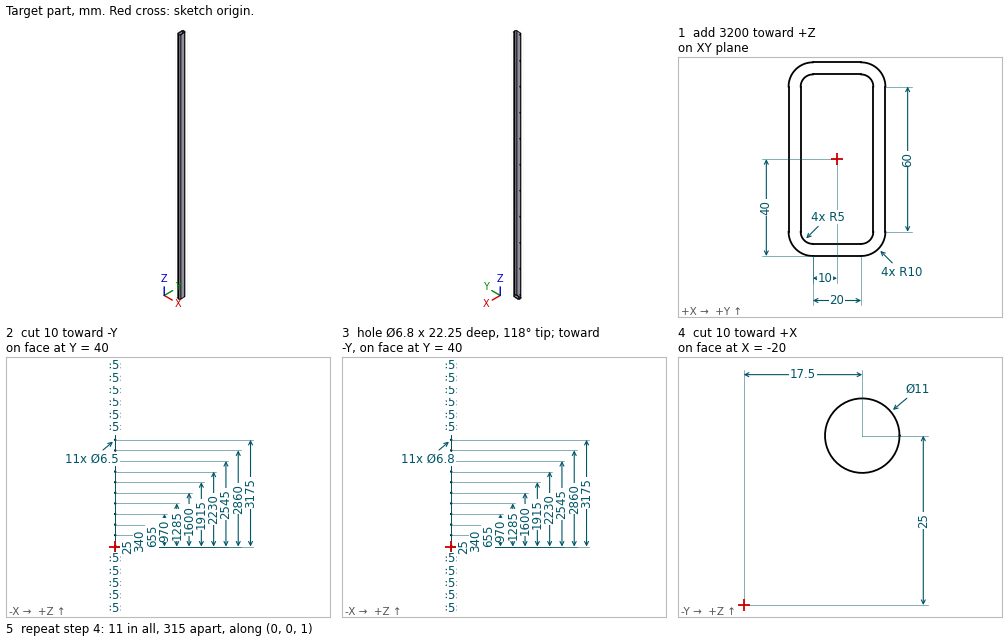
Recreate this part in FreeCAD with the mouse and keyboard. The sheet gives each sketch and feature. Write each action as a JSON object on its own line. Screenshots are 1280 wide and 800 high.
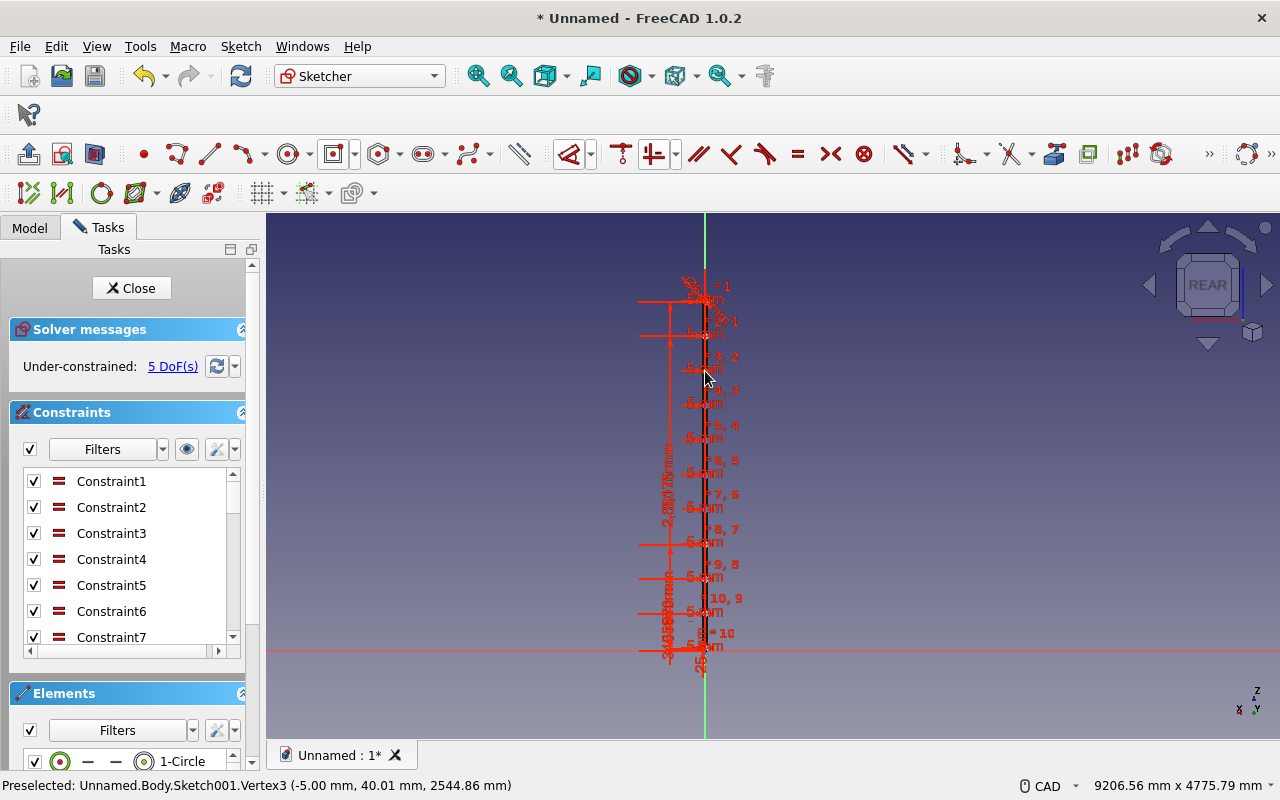
{"action": "key", "text": "i"}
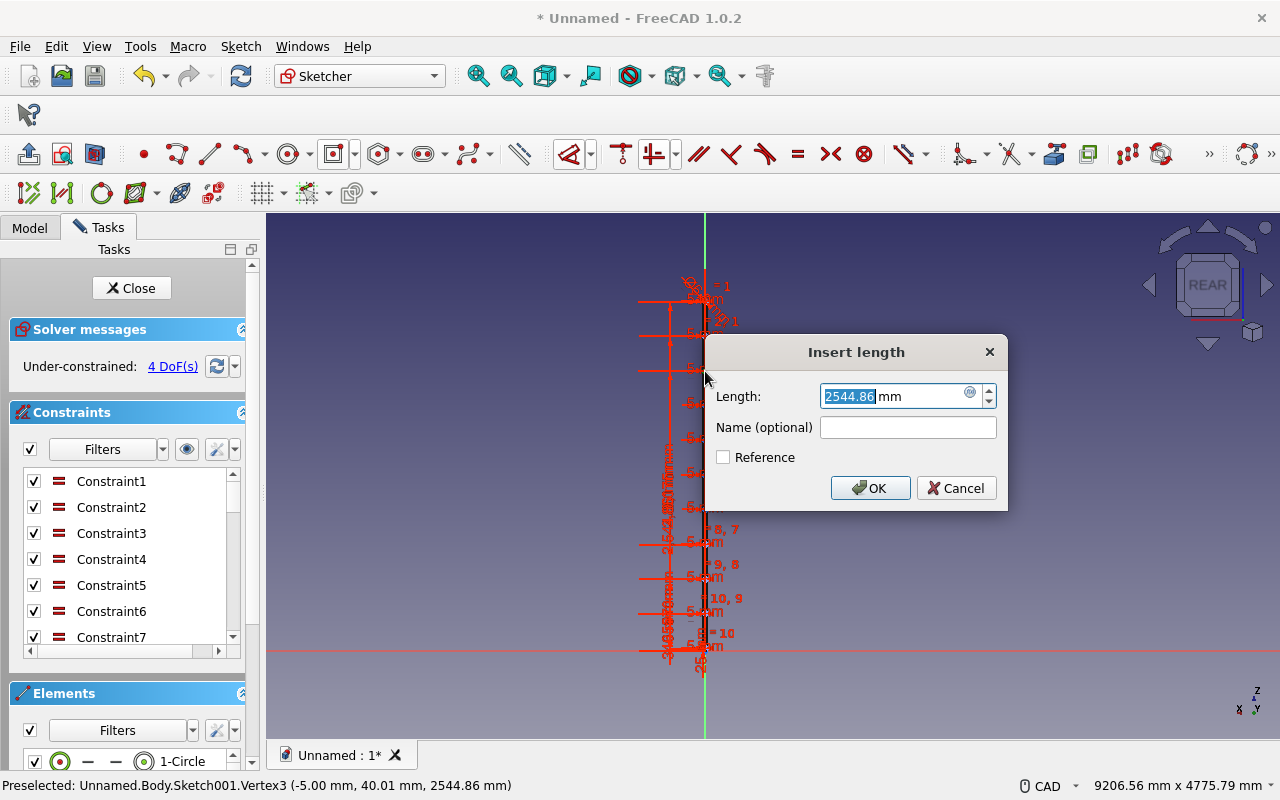
{"action": "type", "text": "2545"}
{"action": "key", "text": "Return"}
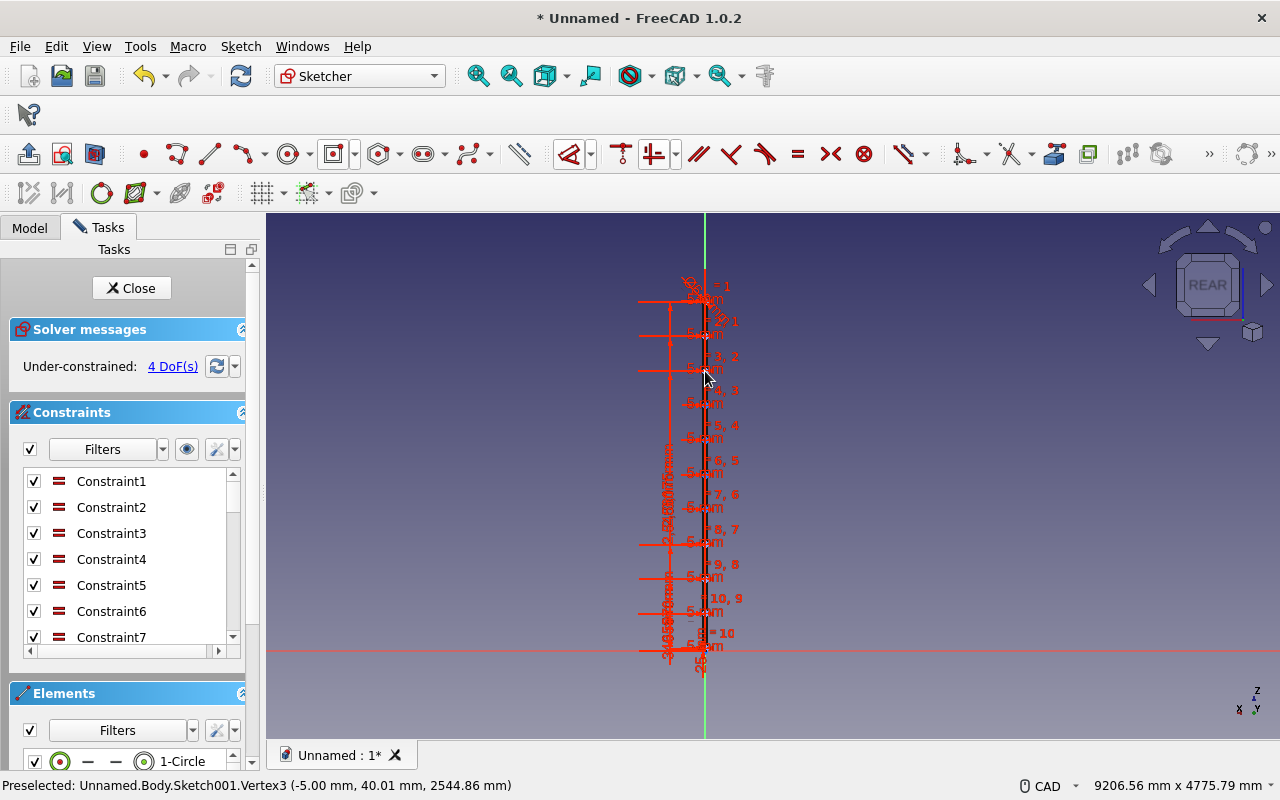
{"action": "left_click", "coordinate": [705, 406]}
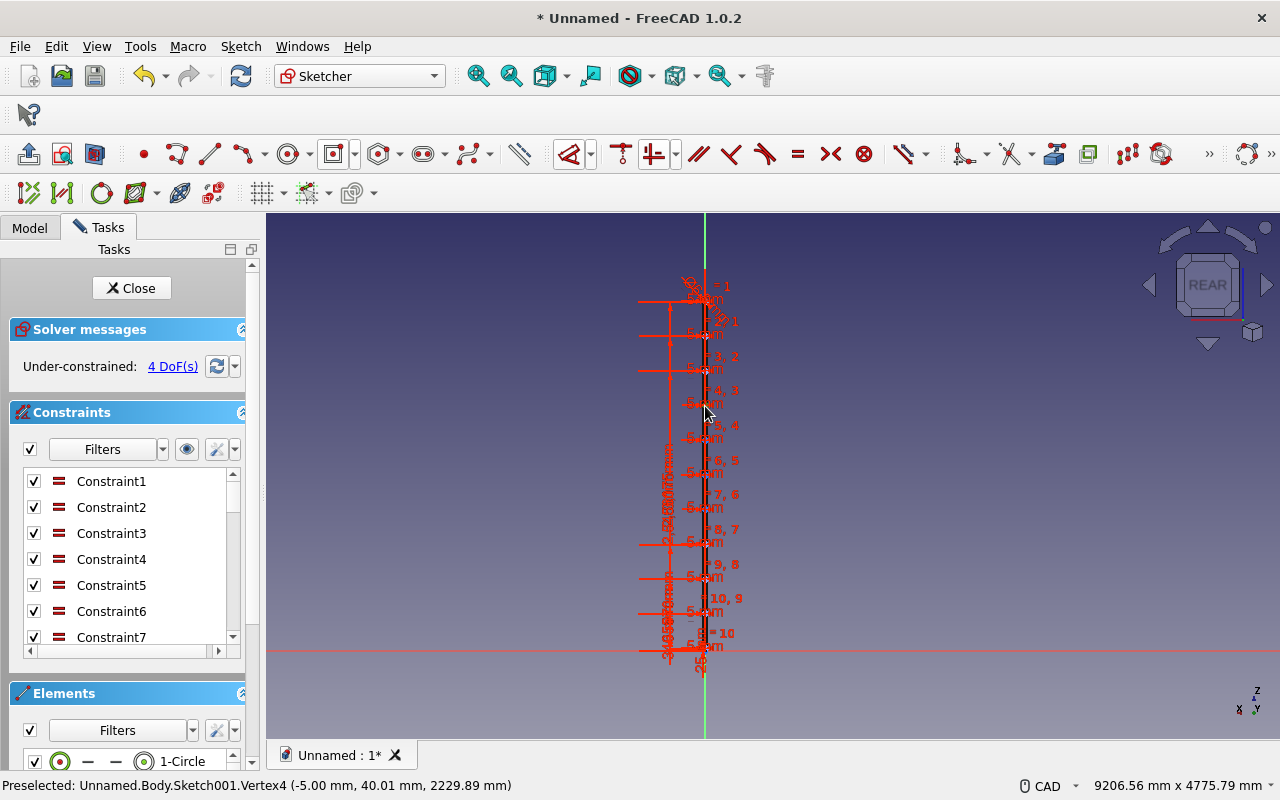
{"action": "left_click", "coordinate": [590, 154]}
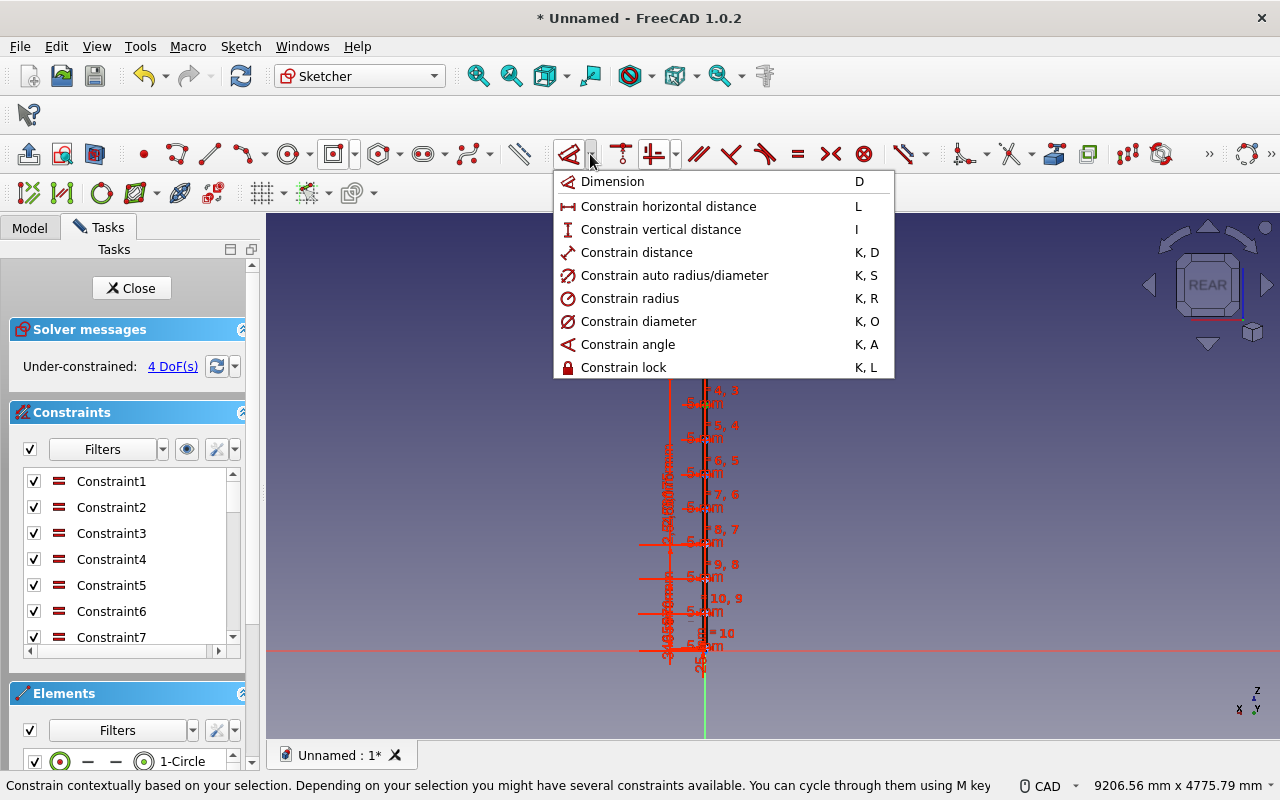
{"action": "left_click", "coordinate": [724, 230]}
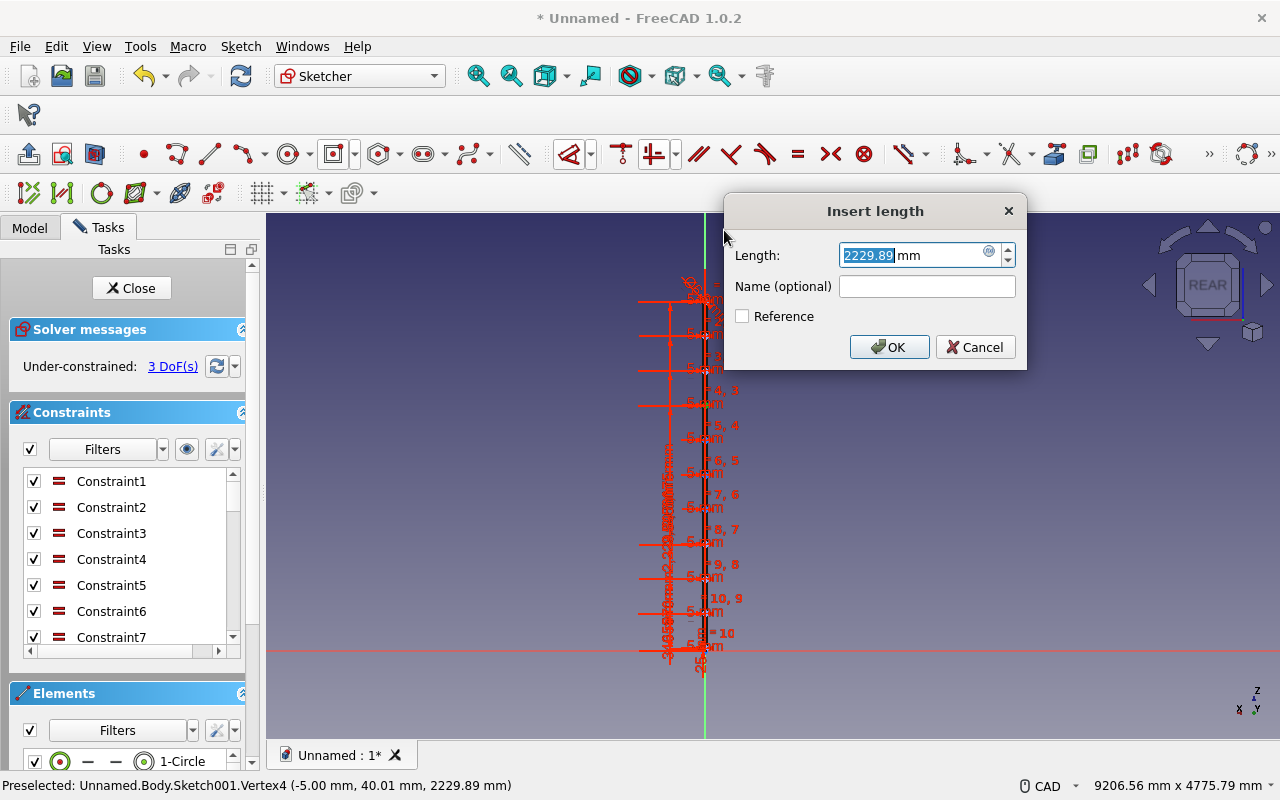
{"action": "type", "text": "2230"}
{"action": "key", "text": "Return"}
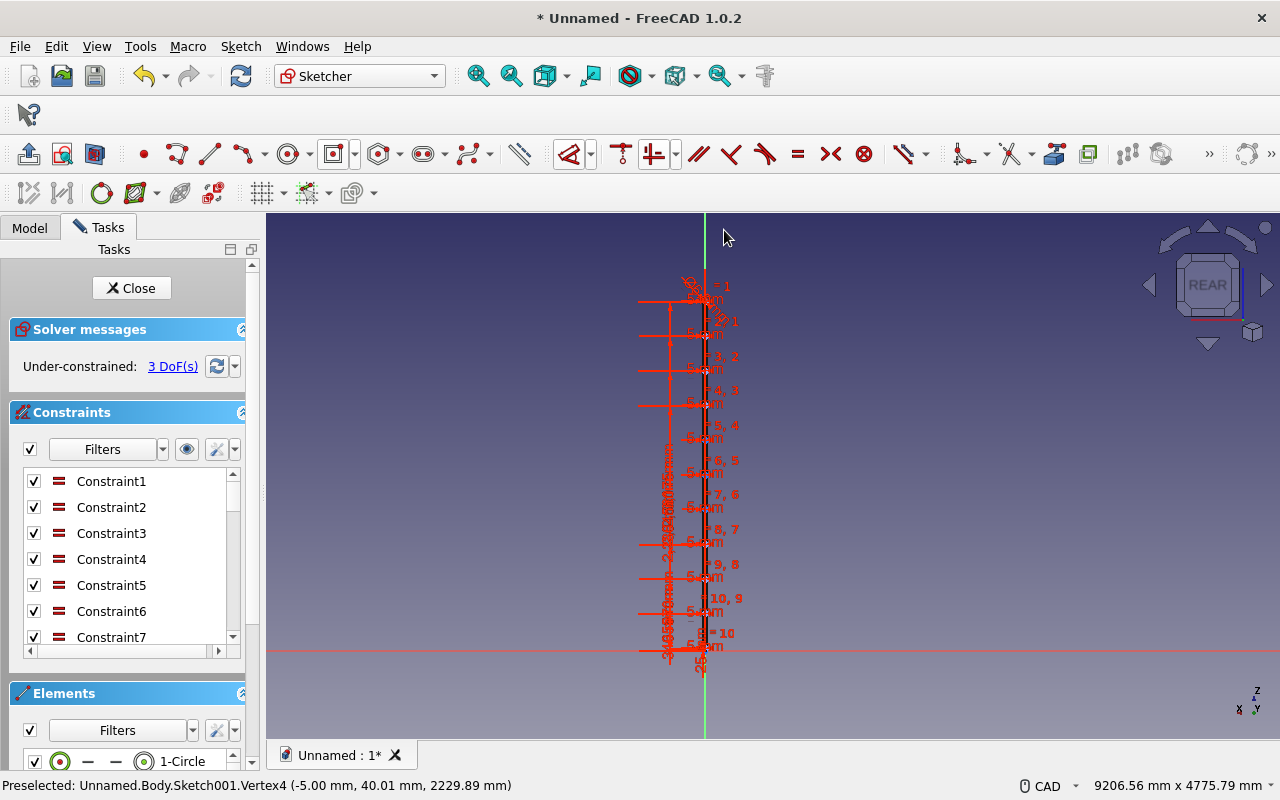
{"action": "left_click", "coordinate": [705, 441]}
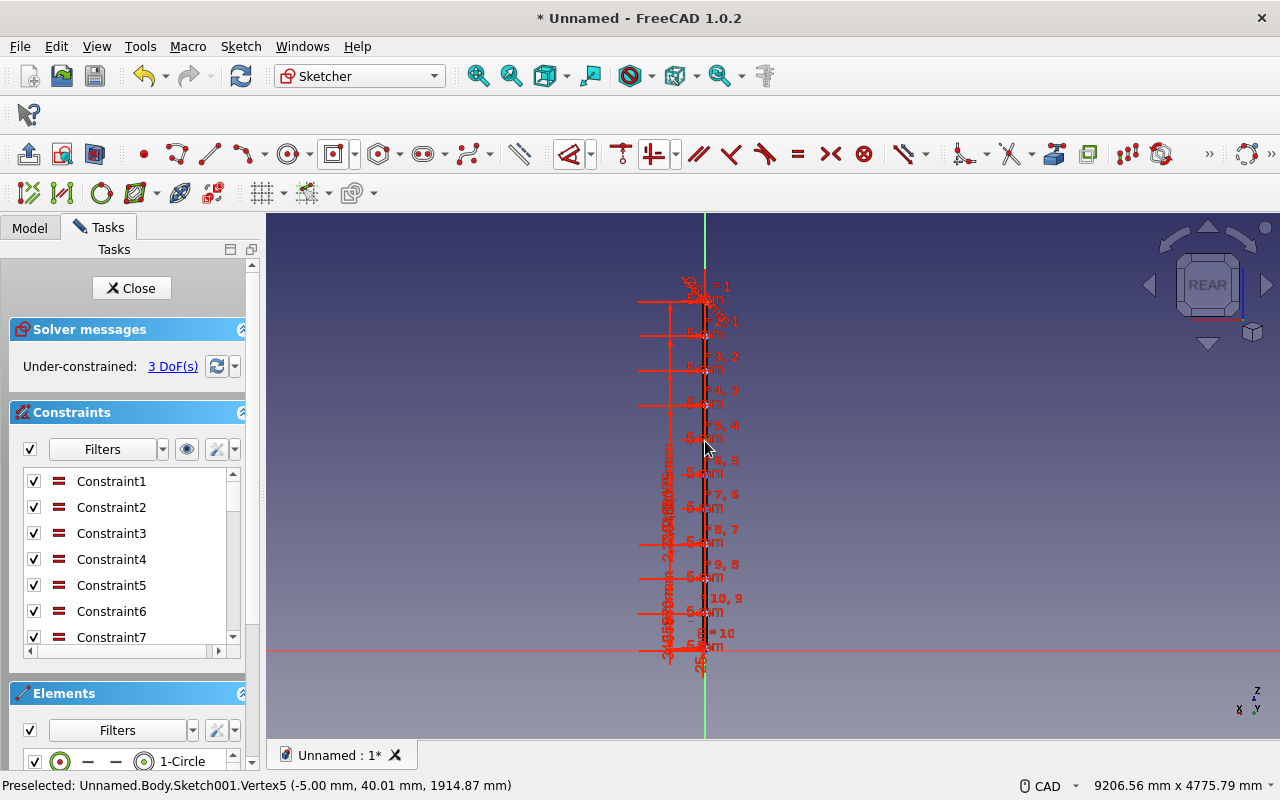
{"action": "key", "text": "i"}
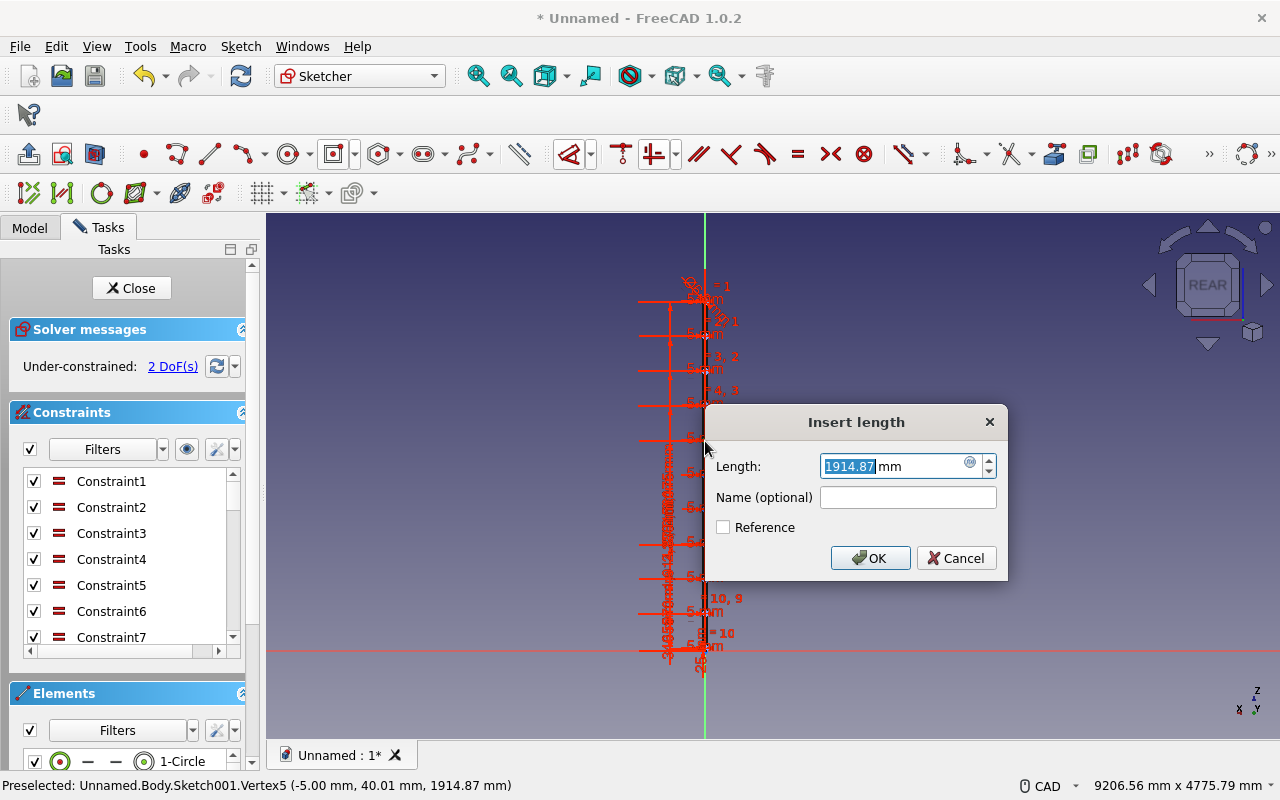
{"action": "type", "text": "1915"}
{"action": "key", "text": "Return"}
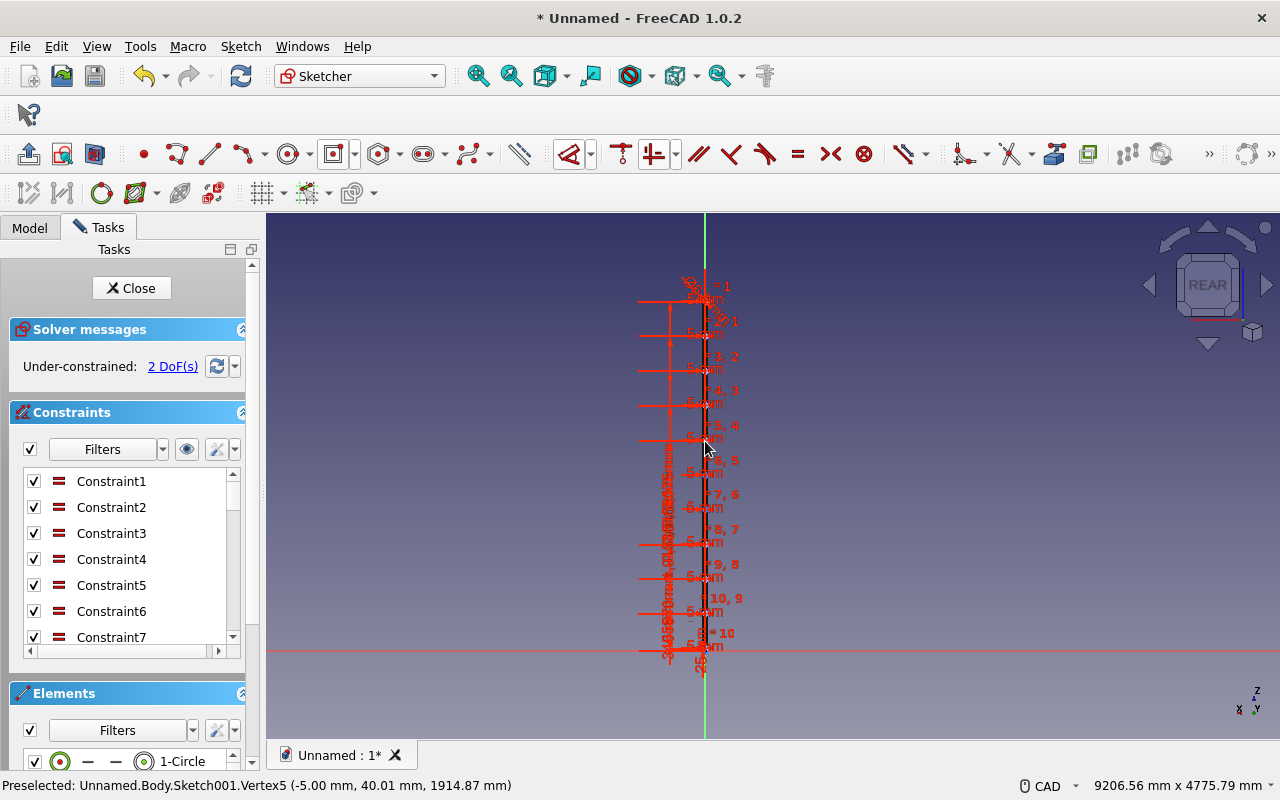
{"action": "left_click", "coordinate": [705, 475]}